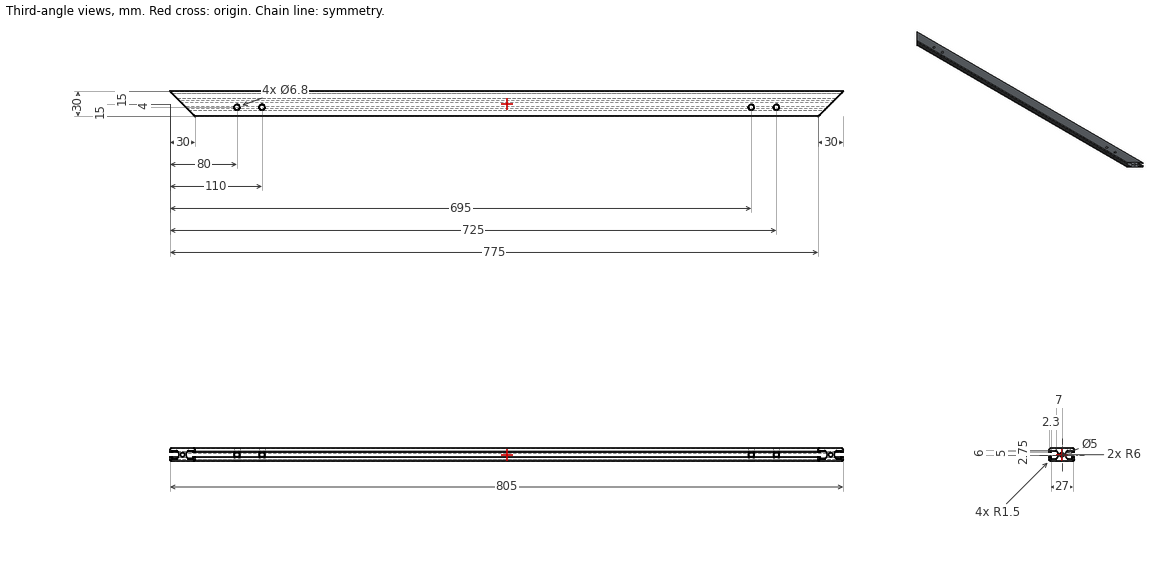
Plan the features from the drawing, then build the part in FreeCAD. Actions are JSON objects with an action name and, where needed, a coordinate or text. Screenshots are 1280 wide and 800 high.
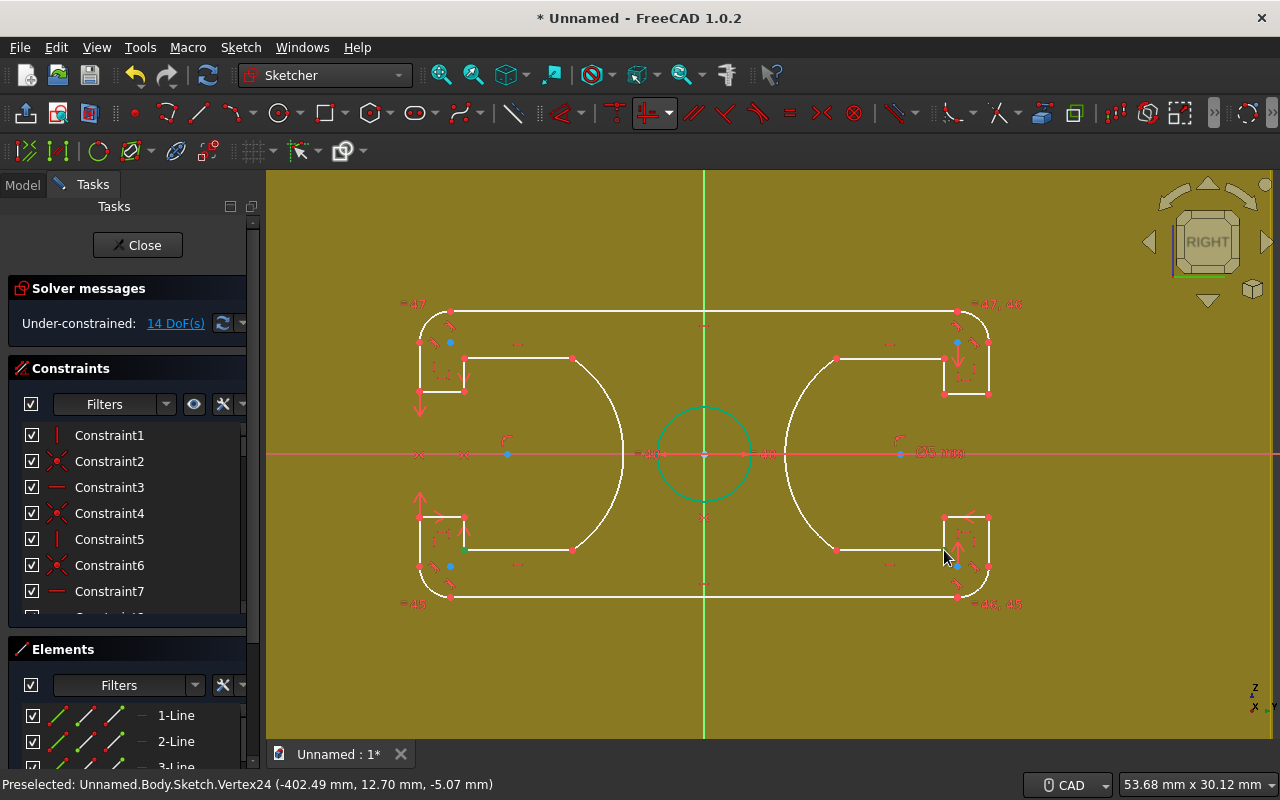
{"action": "left_click", "coordinate": [704, 674]}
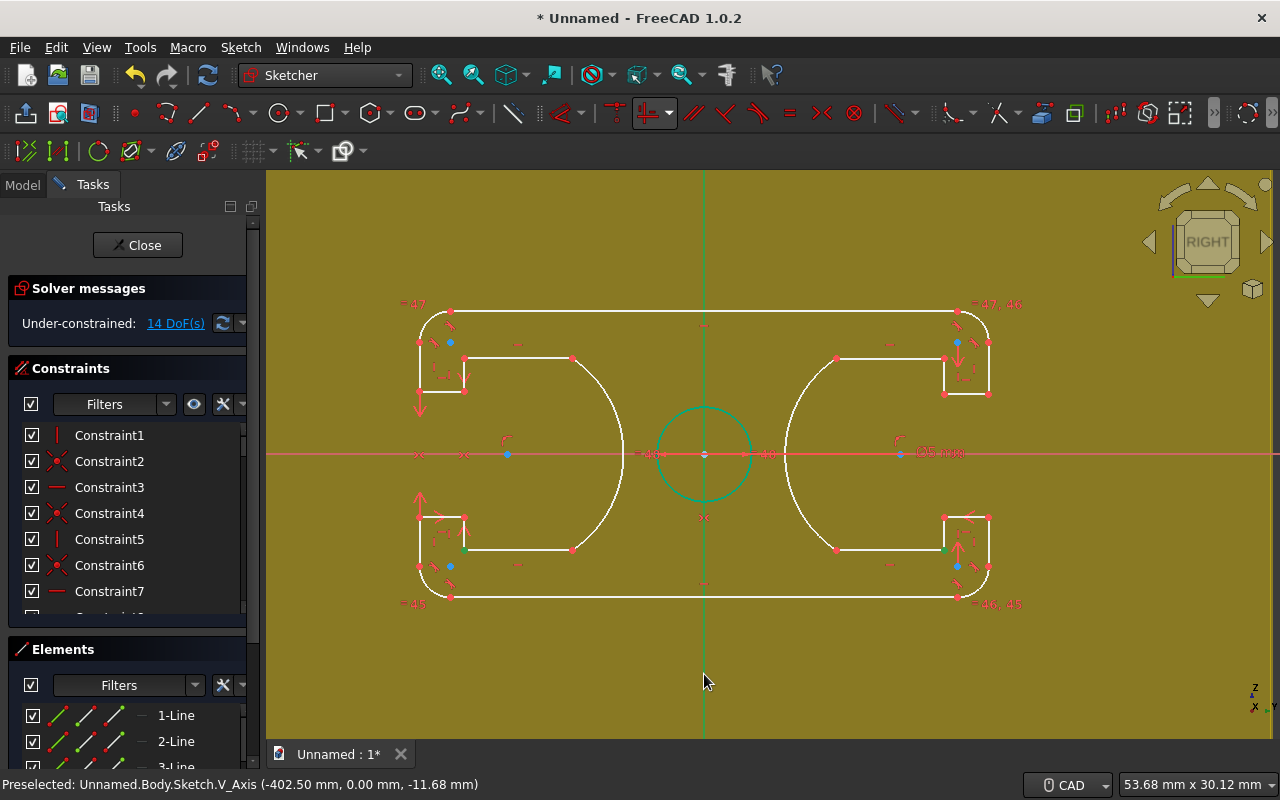
{"action": "left_click", "coordinate": [822, 114]}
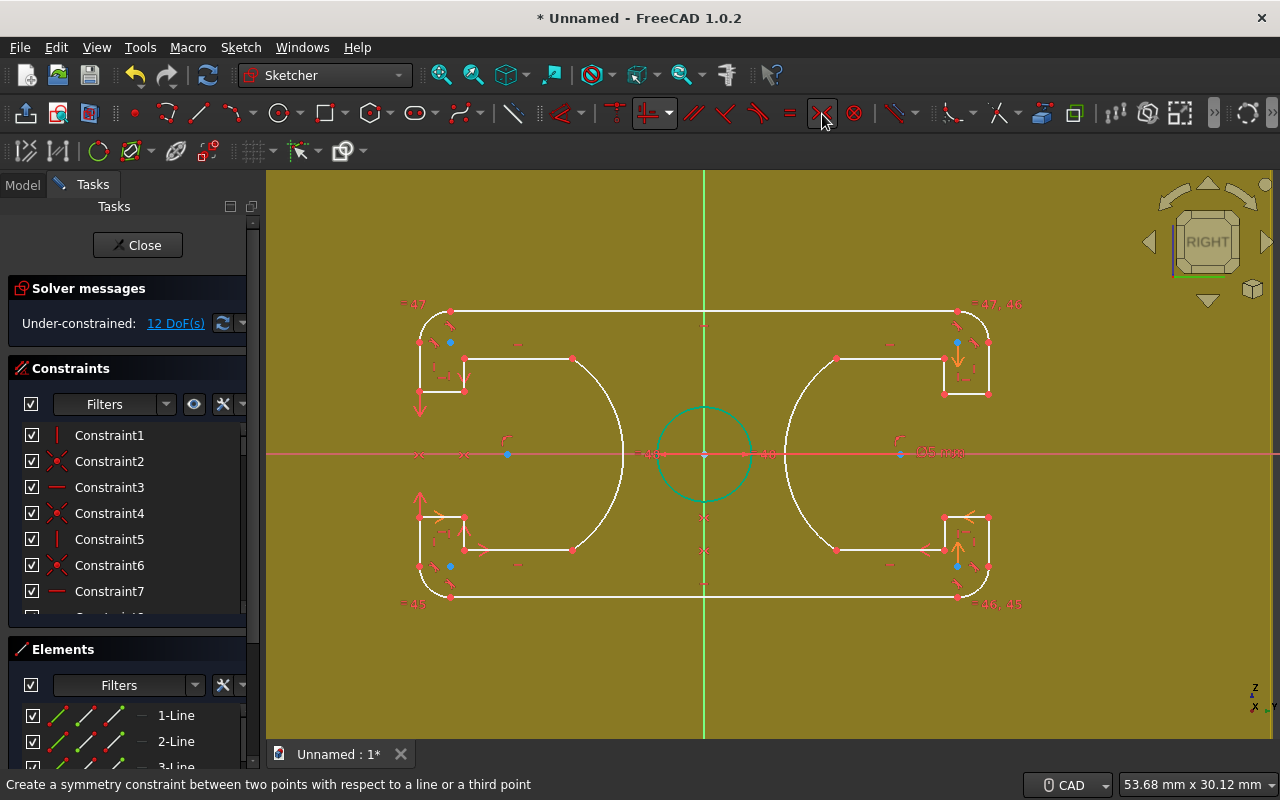
{"action": "left_click", "coordinate": [572, 359]}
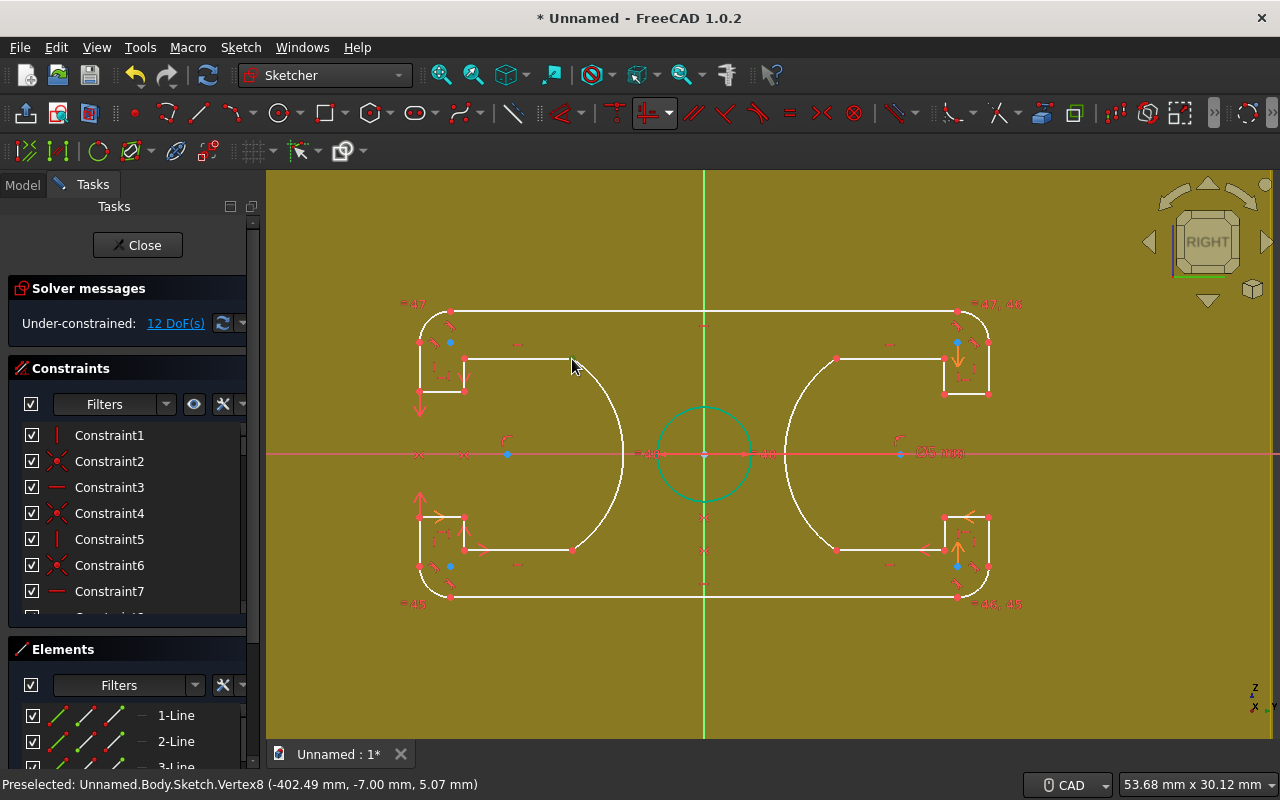
{"action": "left_click", "coordinate": [836, 359]}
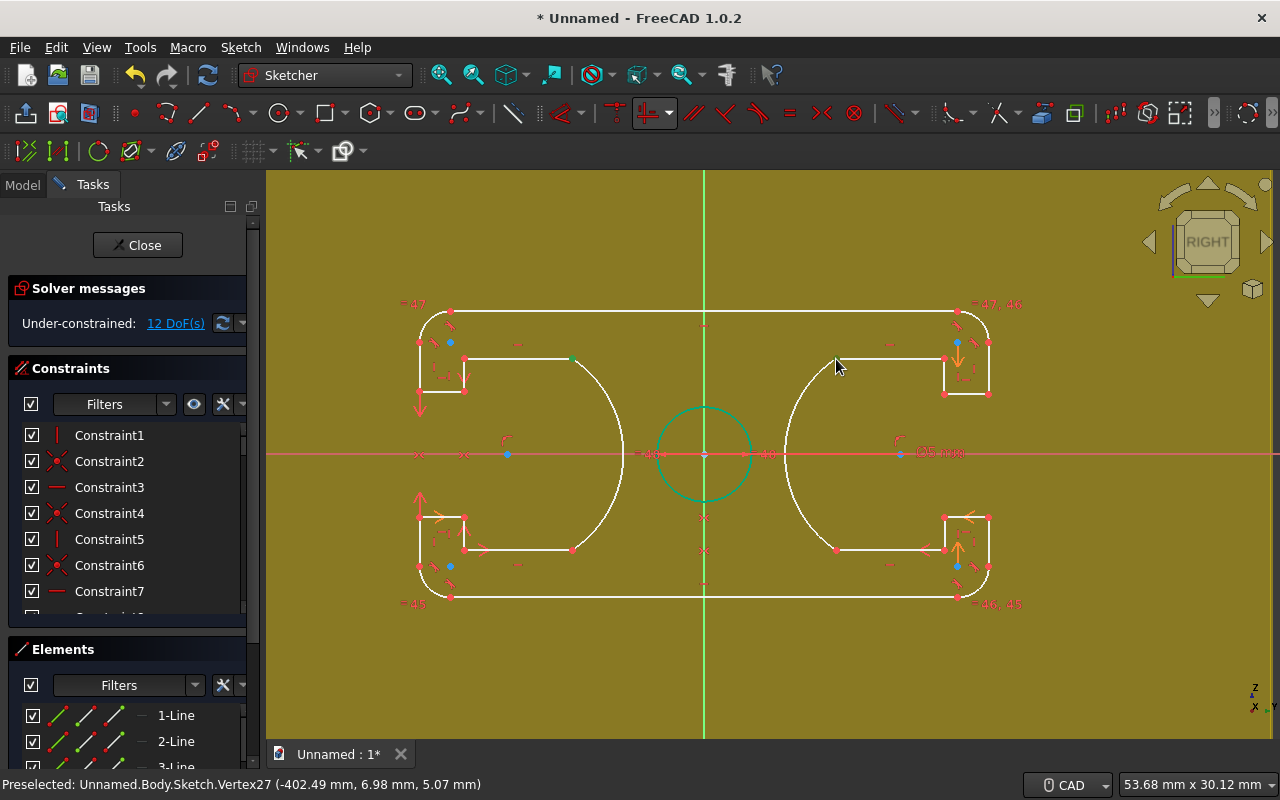
{"action": "left_click", "coordinate": [704, 674]}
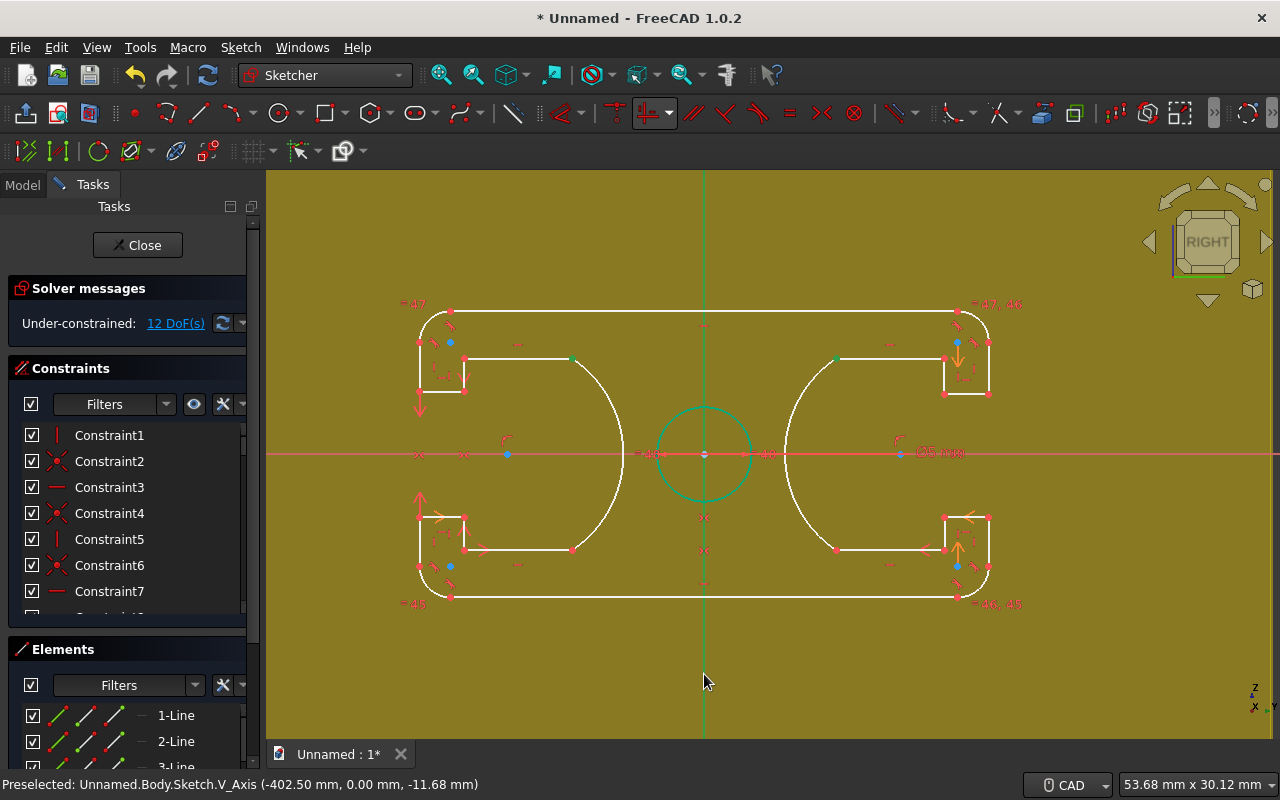
{"action": "left_click", "coordinate": [822, 114]}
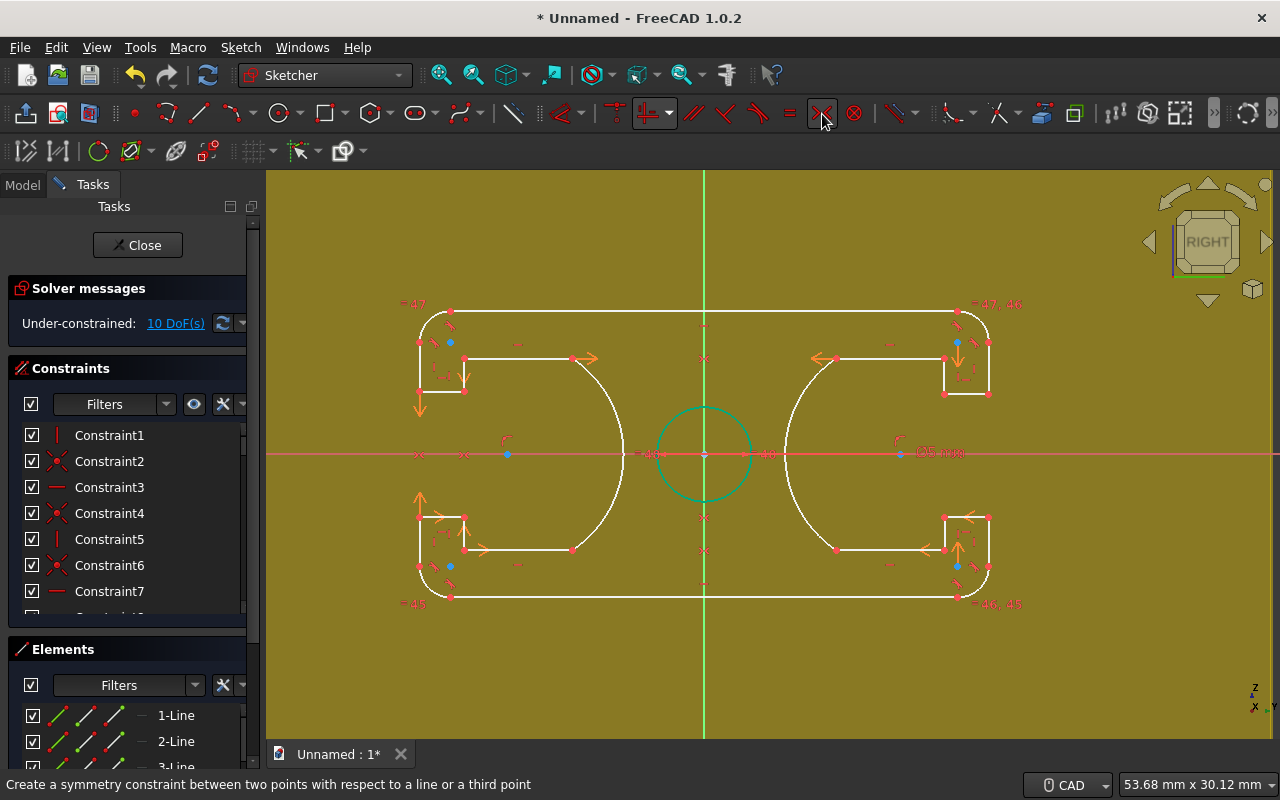
{"action": "left_click", "coordinate": [464, 392]}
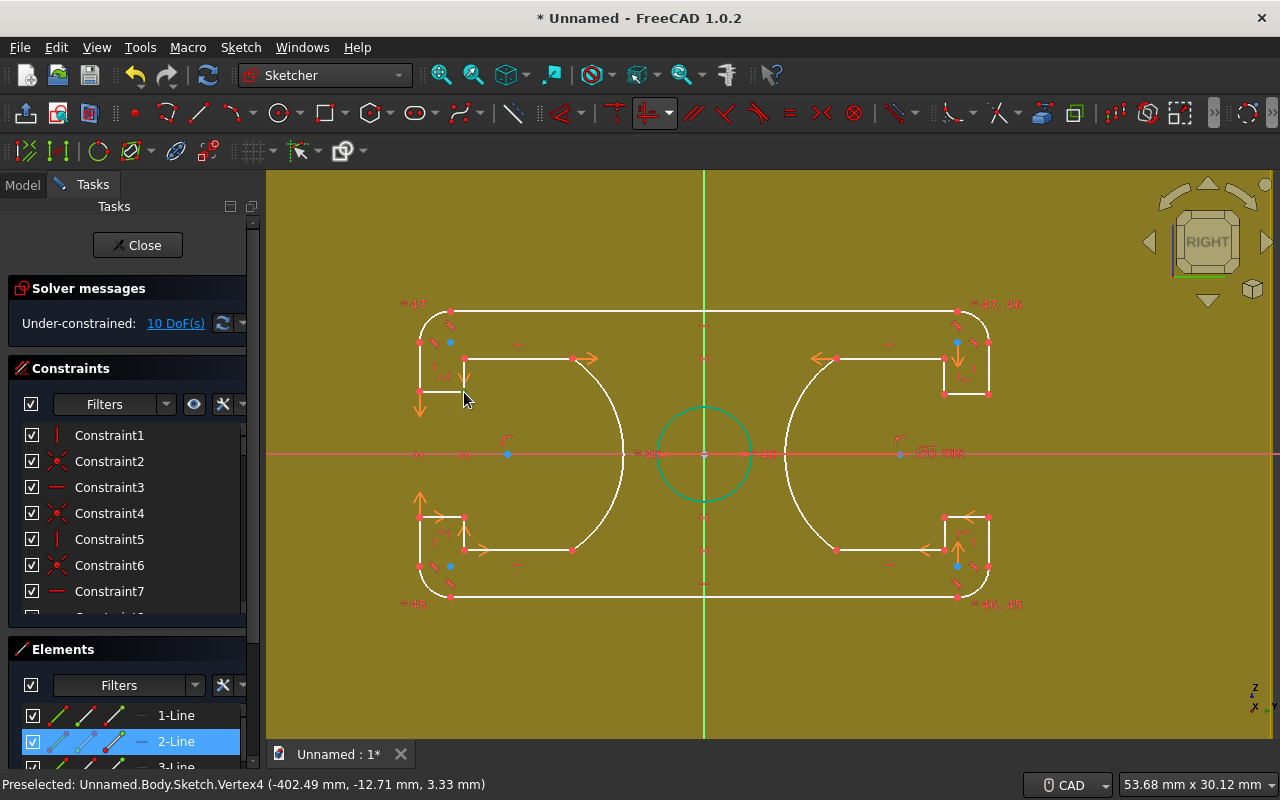
{"action": "left_click", "coordinate": [944, 394]}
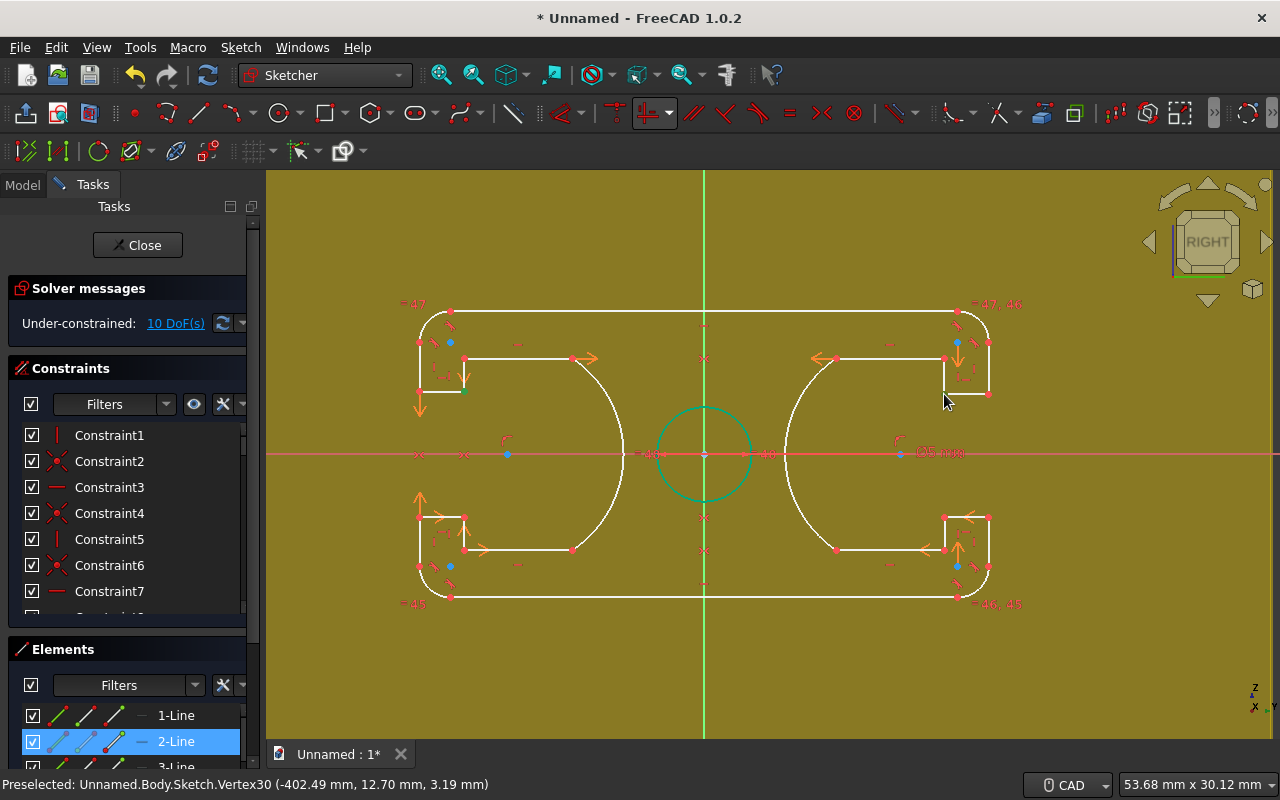
{"action": "left_click", "coordinate": [704, 674]}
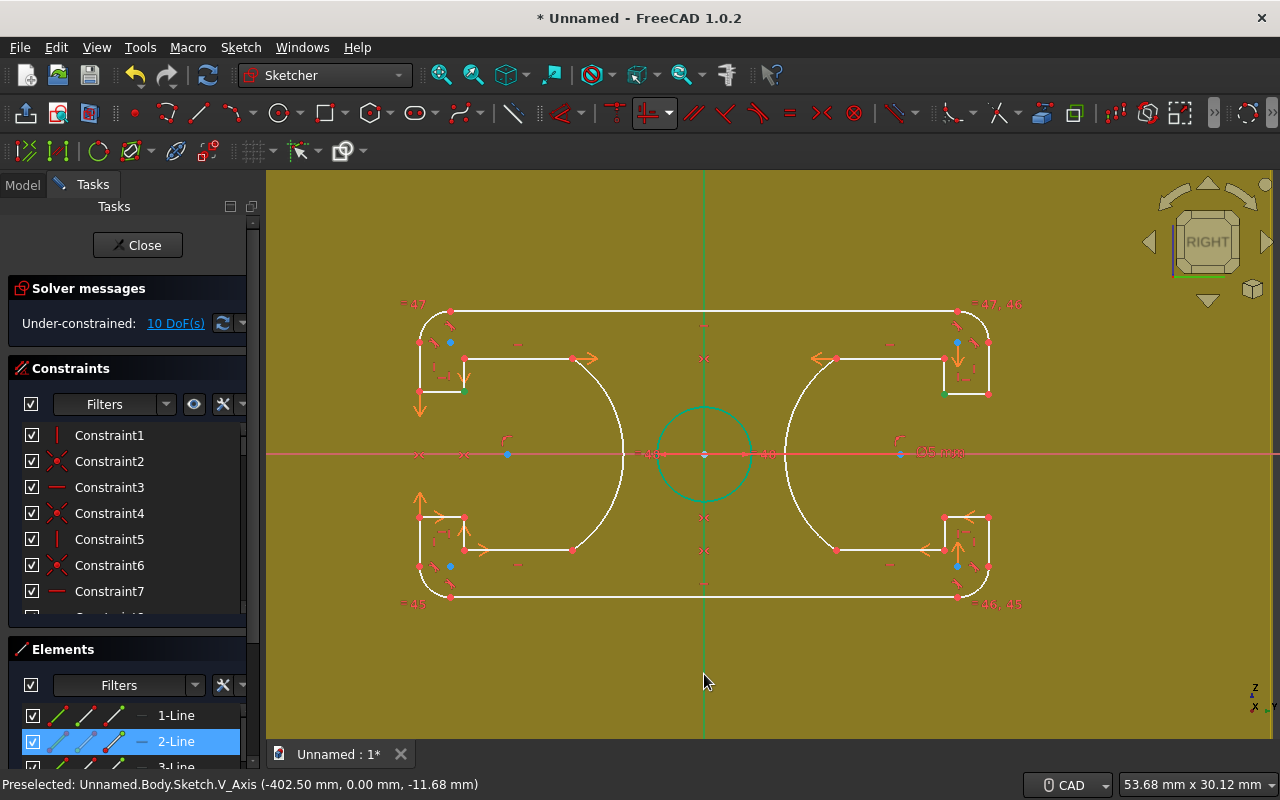
{"action": "left_click", "coordinate": [822, 114]}